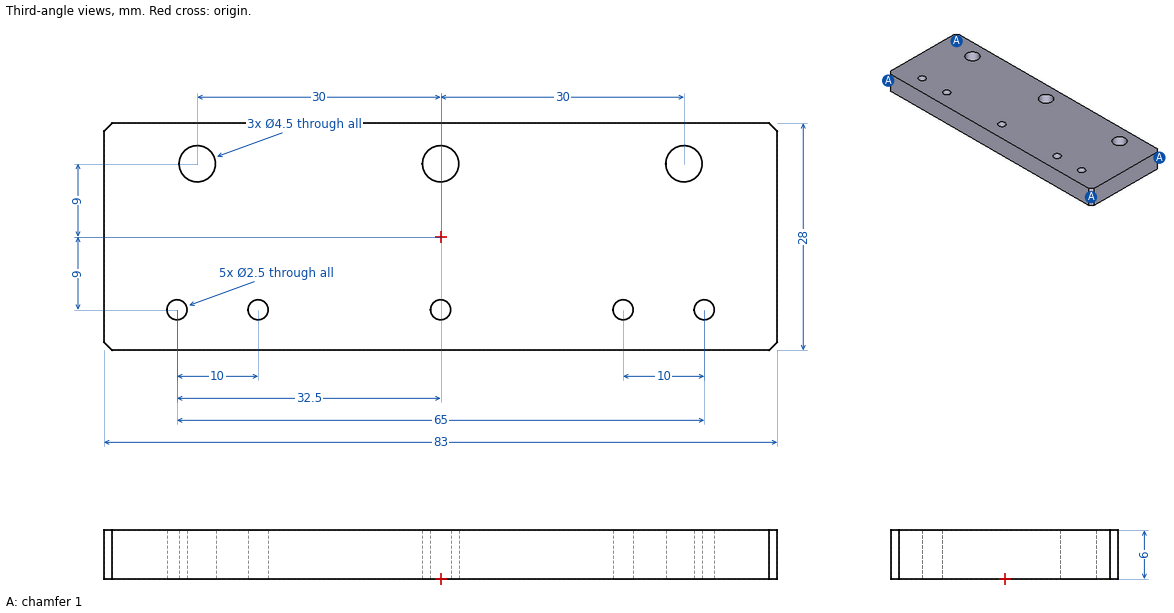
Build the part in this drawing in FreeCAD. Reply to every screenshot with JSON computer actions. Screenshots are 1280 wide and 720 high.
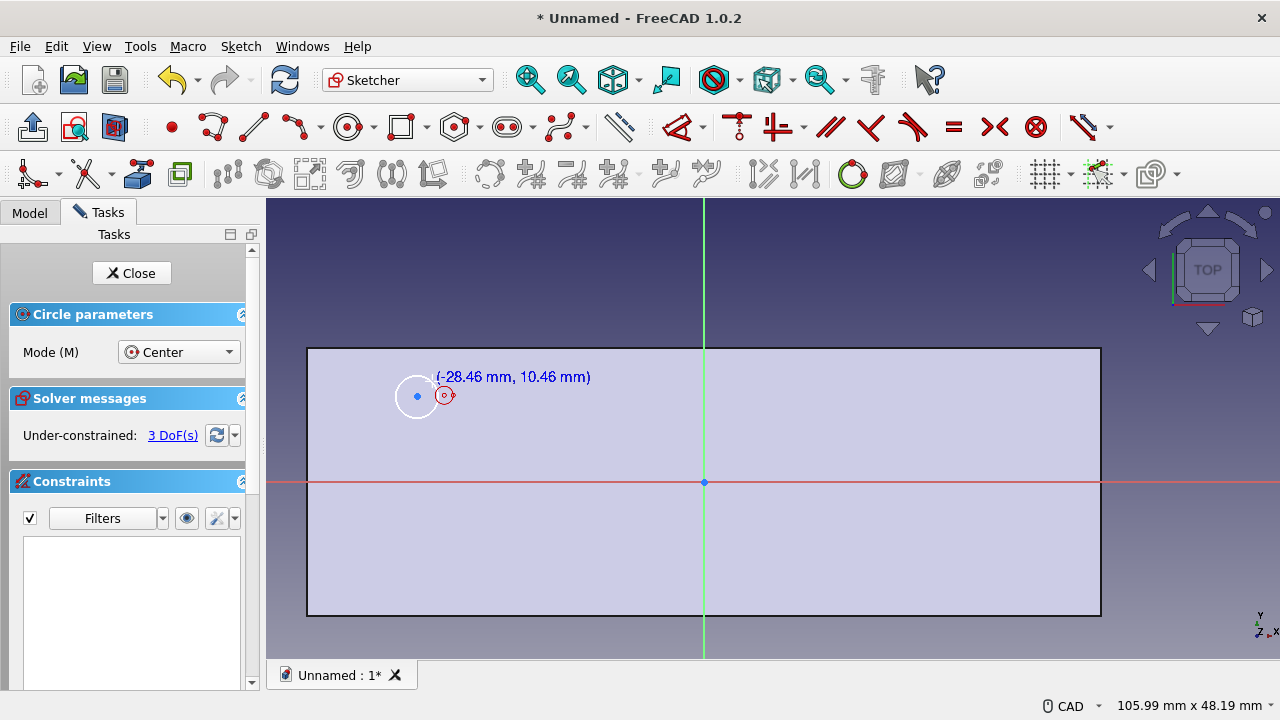
{"action": "left_click", "coordinate": [704, 396]}
{"action": "left_click", "coordinate": [720, 381]}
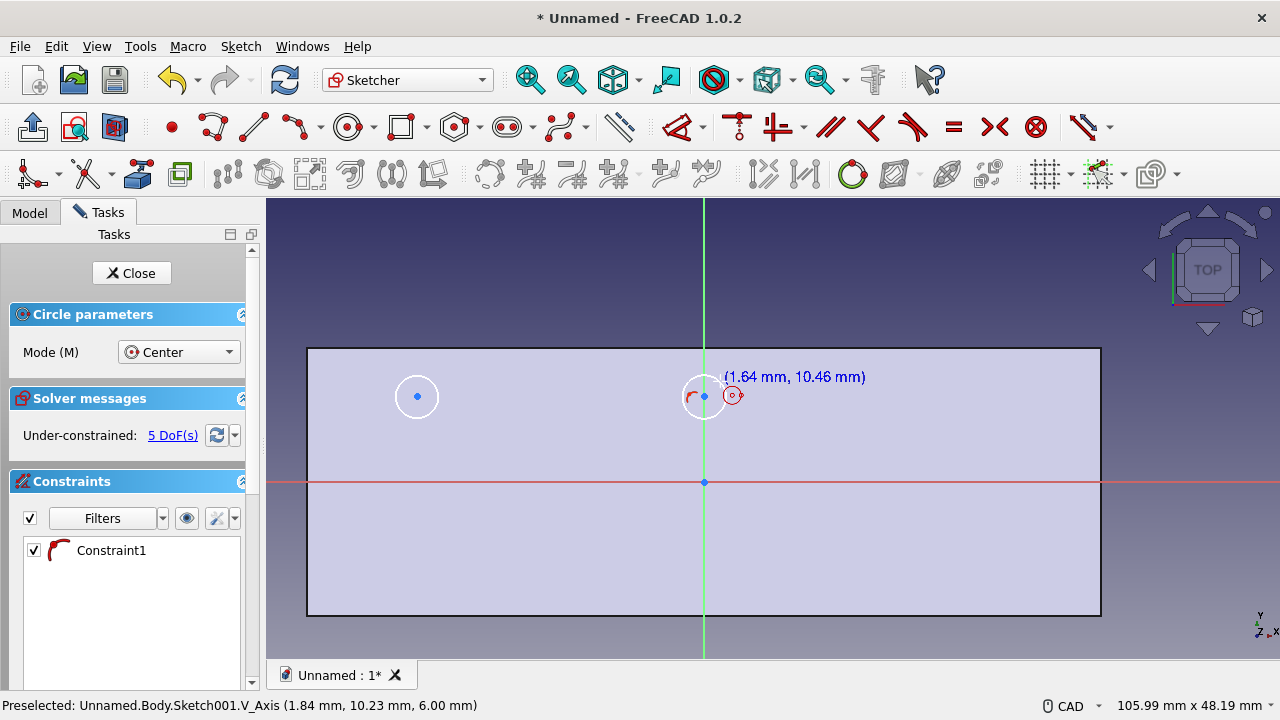
{"action": "left_click", "coordinate": [991, 396]}
{"action": "left_click", "coordinate": [1007, 381]}
{"action": "key", "text": "Escape"}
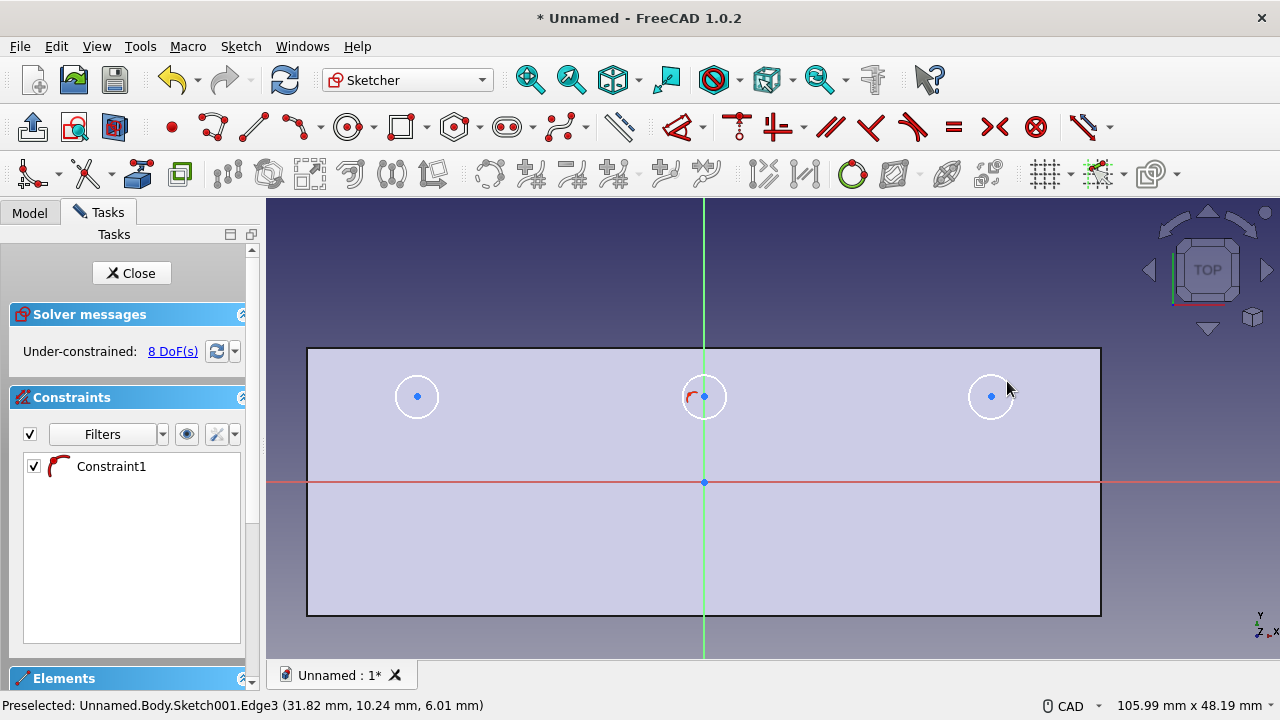
{"action": "left_click", "coordinate": [432, 382]}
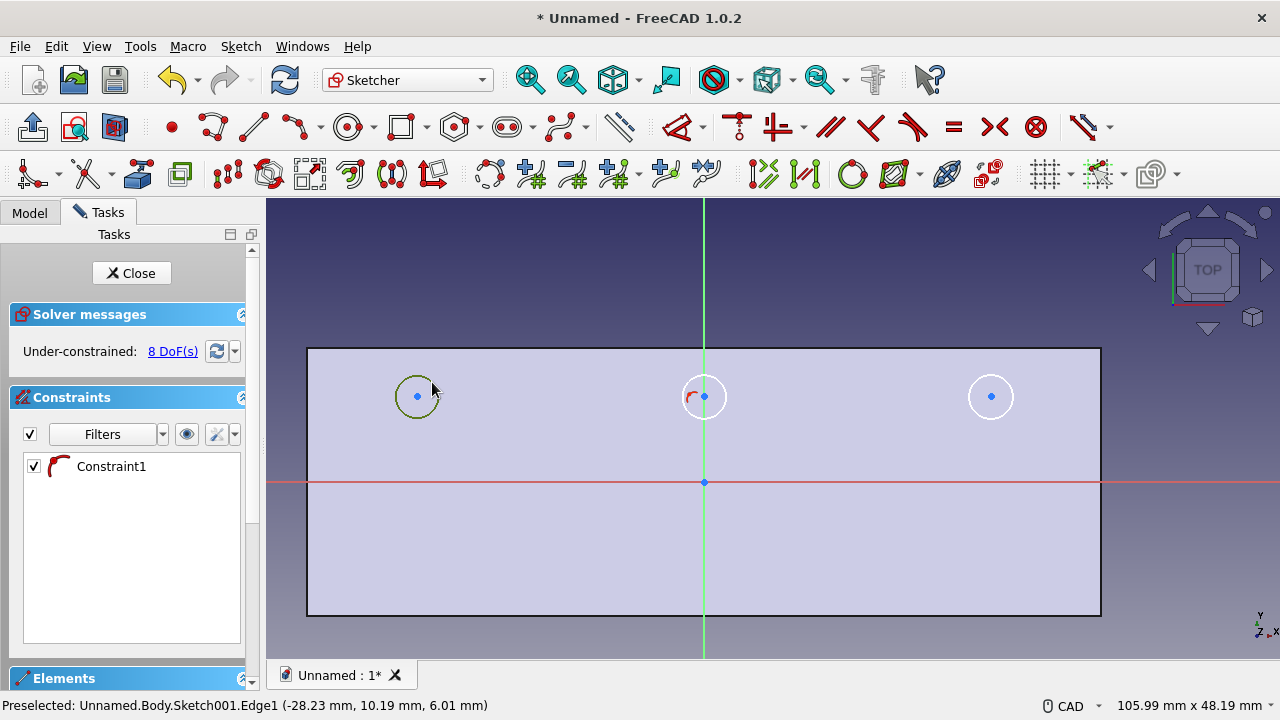
{"action": "left_click", "coordinate": [720, 382]}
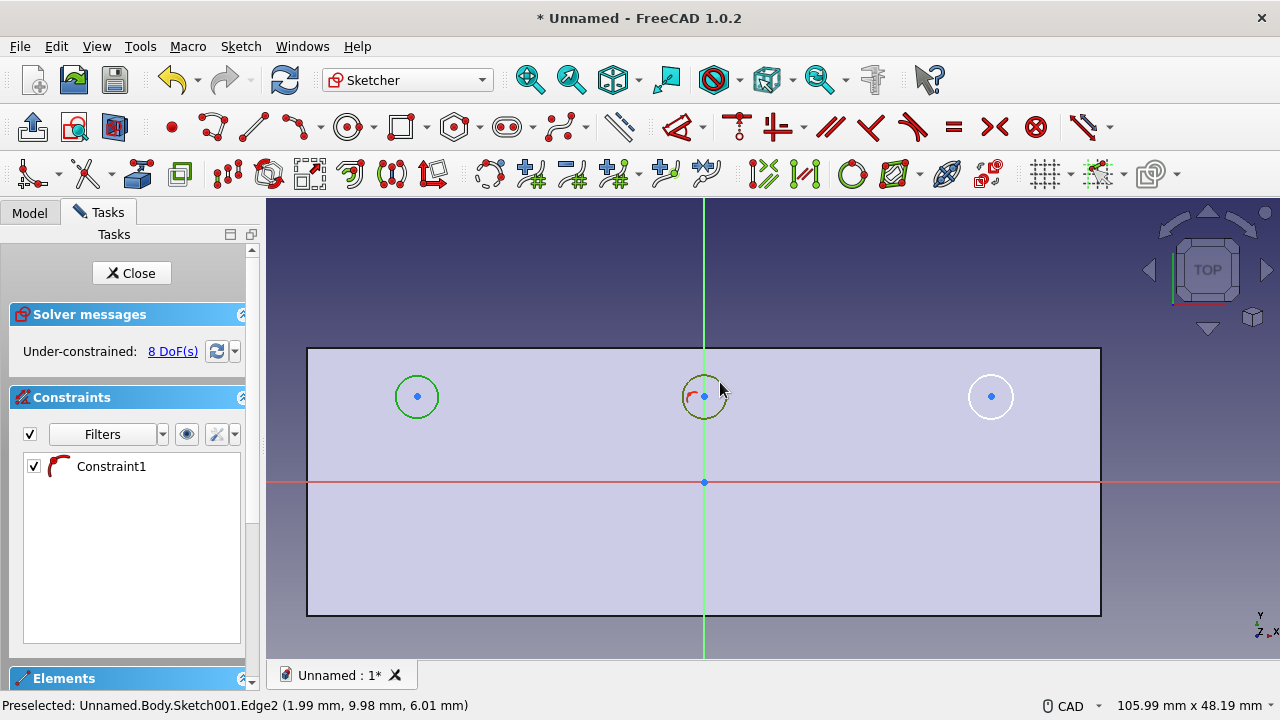
{"action": "left_click", "coordinate": [1006, 381]}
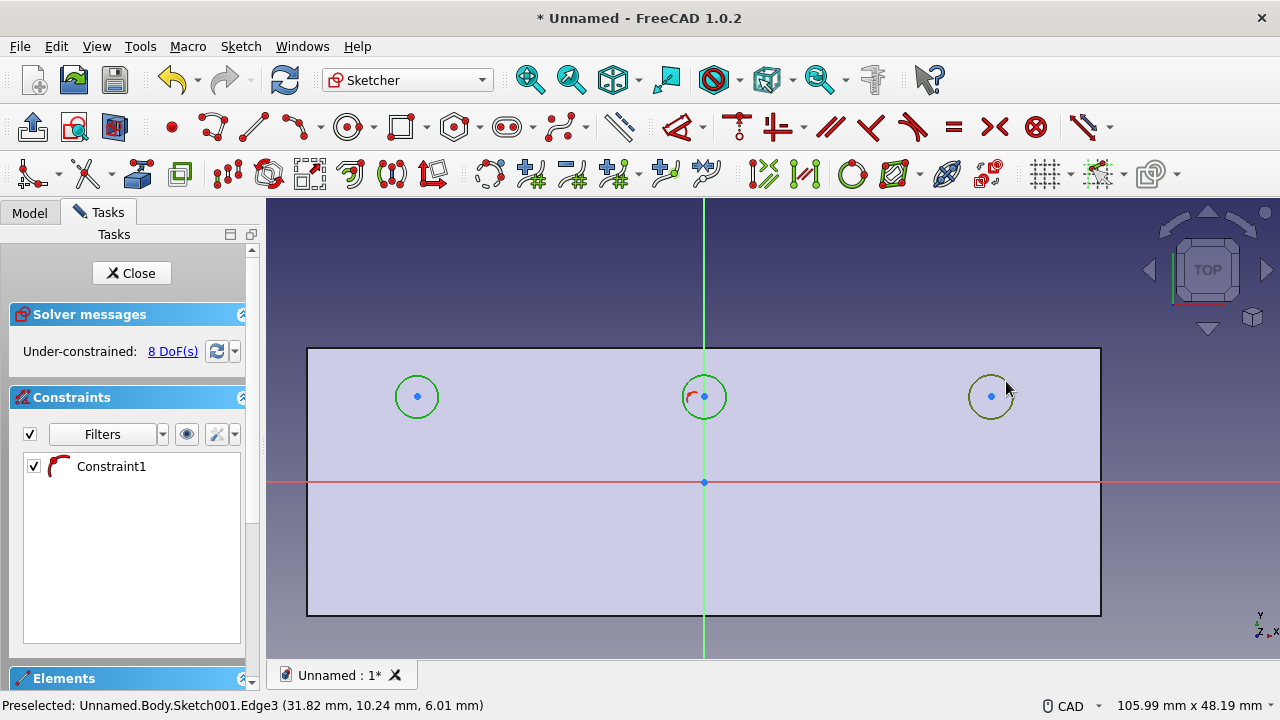
{"action": "left_click", "coordinate": [954, 128]}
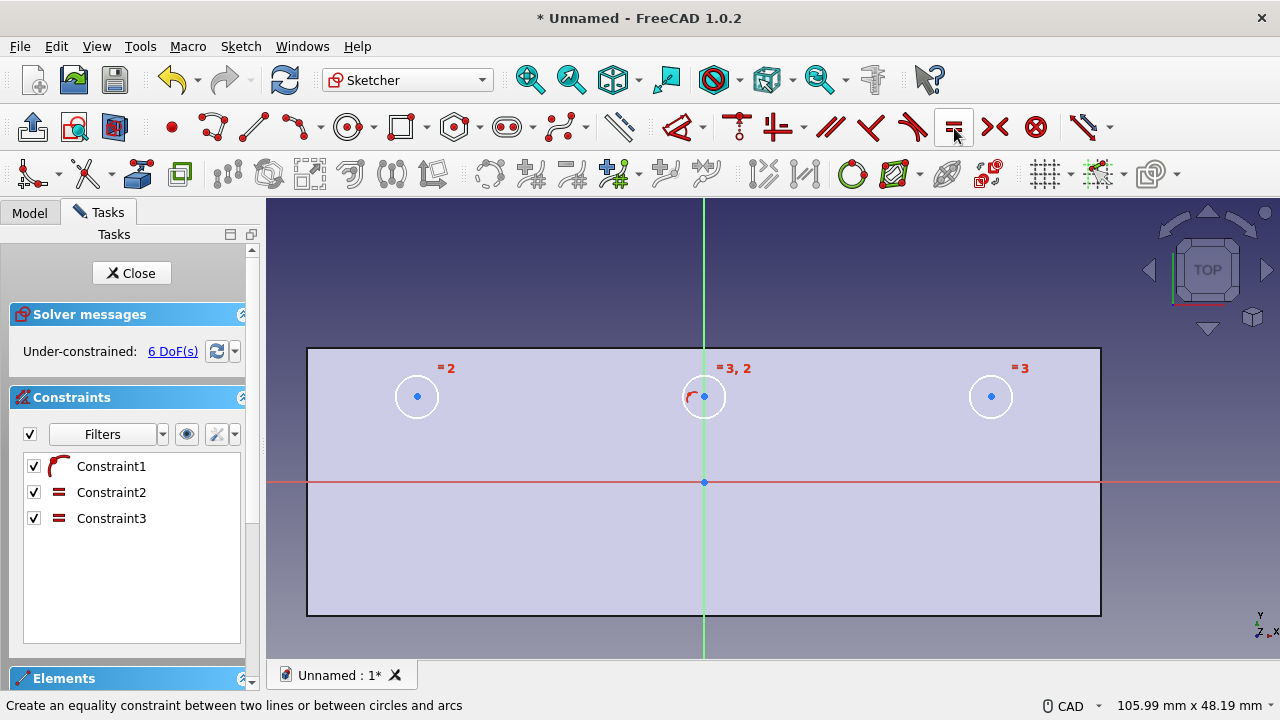
{"action": "key", "text": "d"}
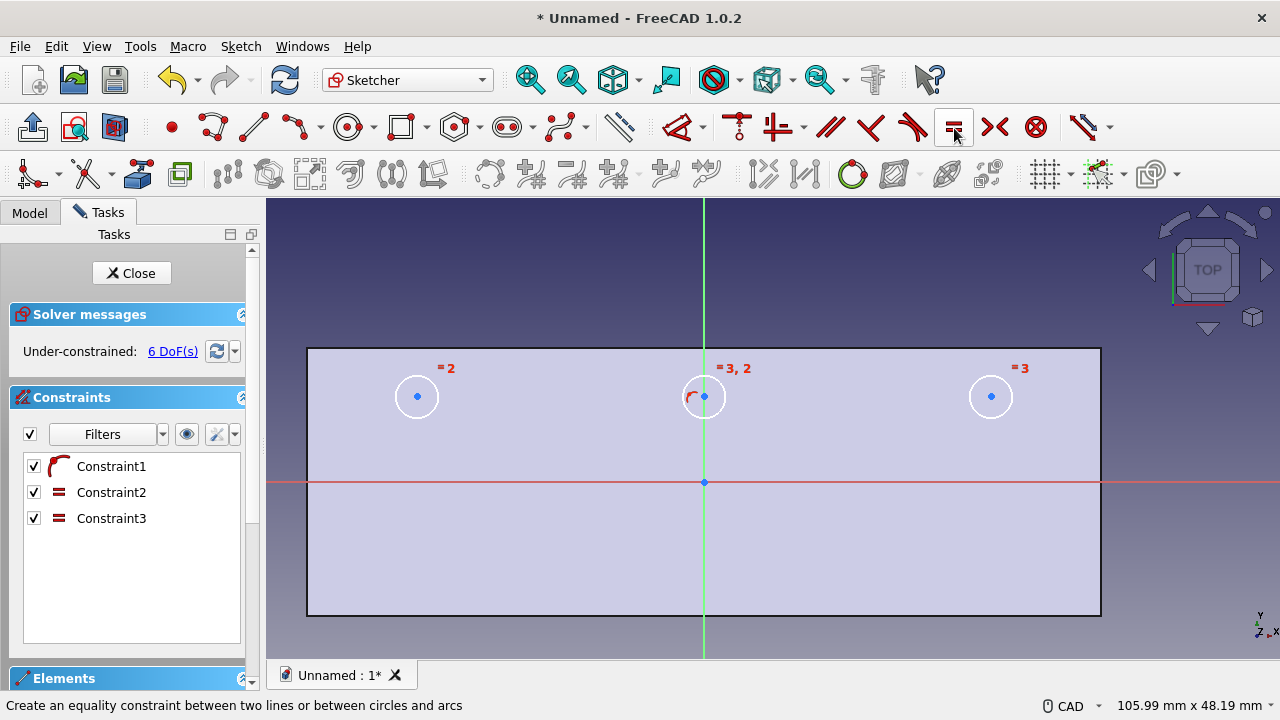
{"action": "left_click", "coordinate": [432, 382]}
{"action": "left_click", "coordinate": [455, 359]}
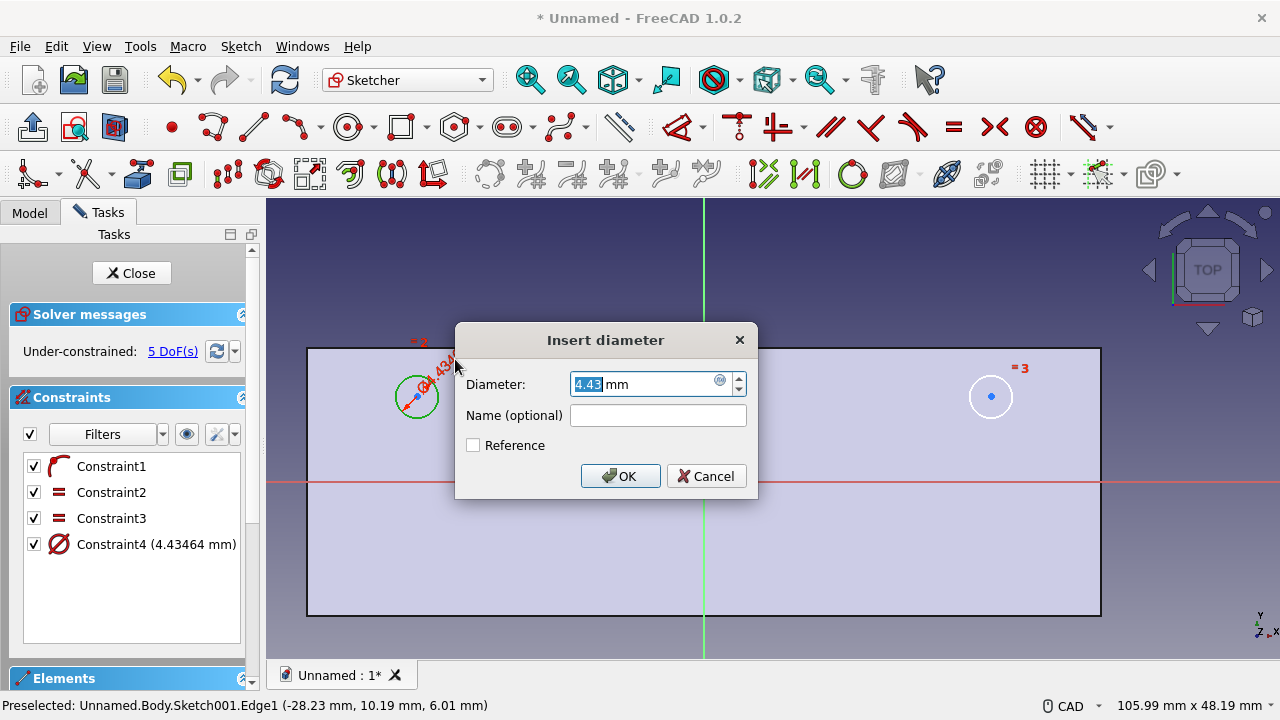
{"action": "type", "text": "4.5"}
{"action": "key", "text": "Return"}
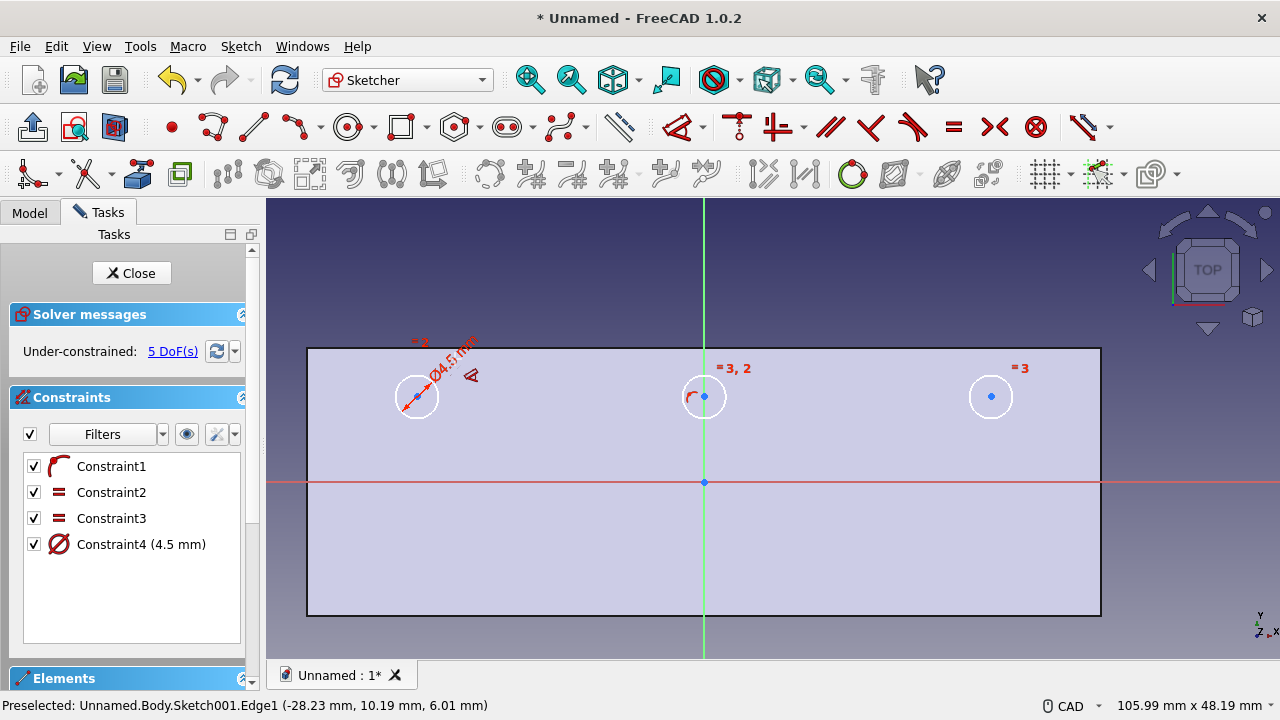
{"action": "left_click", "coordinate": [417, 397]}
{"action": "left_click", "coordinate": [383, 440]}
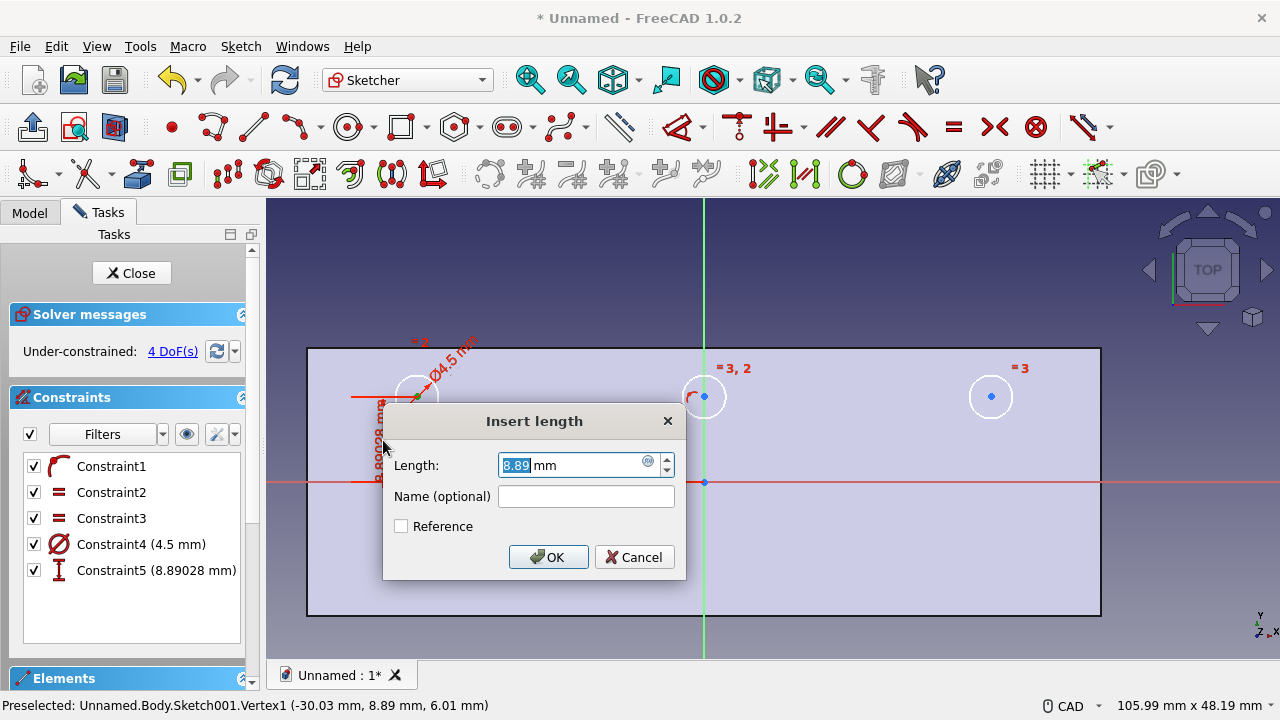
{"action": "type", "text": "9"}
{"action": "key", "text": "Return"}